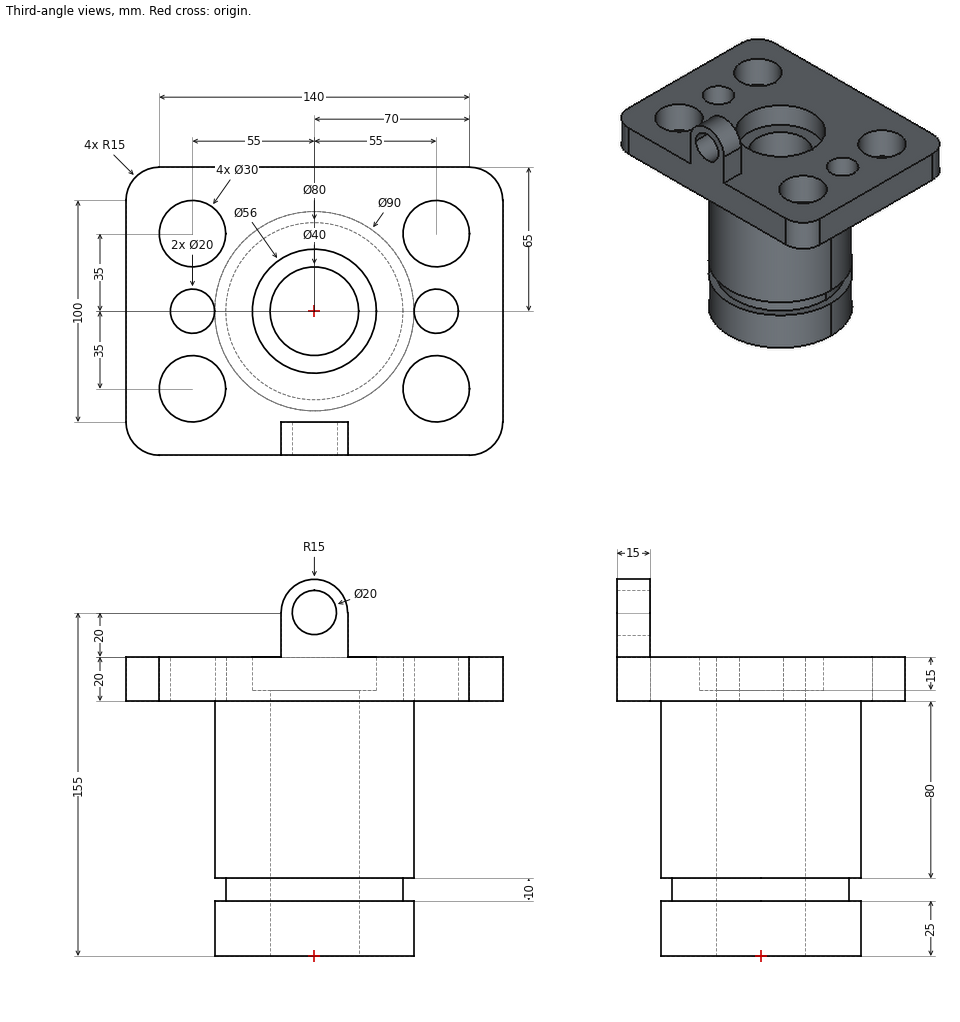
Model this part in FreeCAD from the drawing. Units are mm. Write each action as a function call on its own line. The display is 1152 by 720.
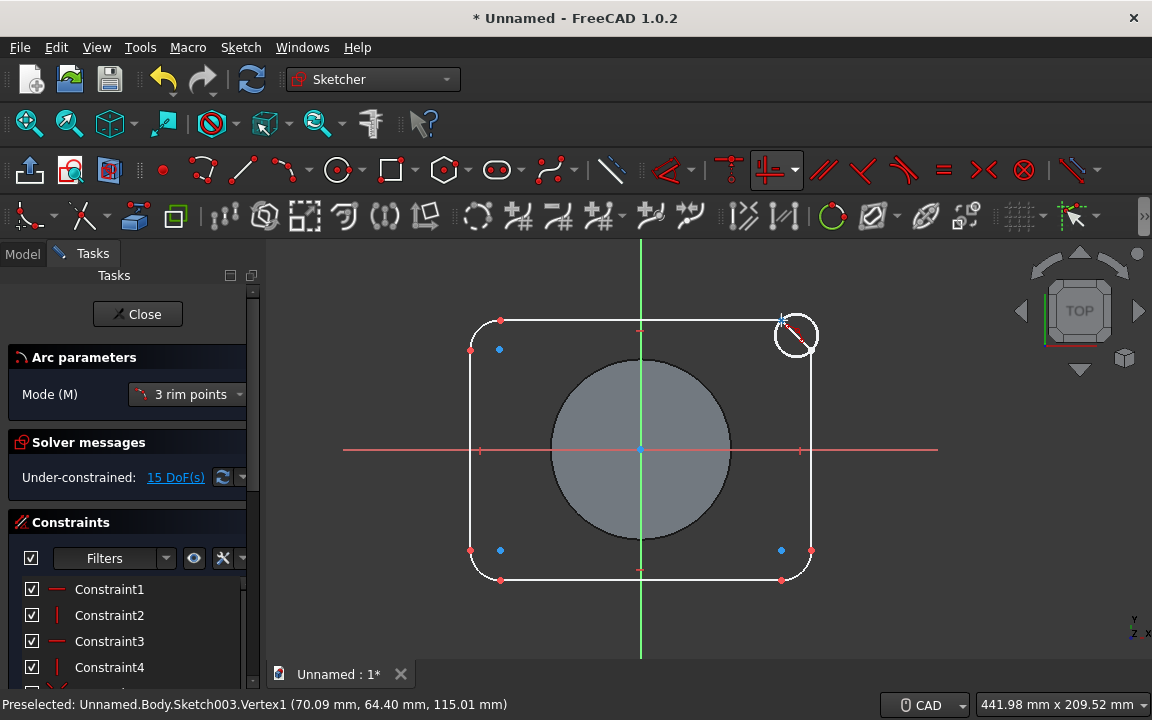
scroll(803, 328, up, 3)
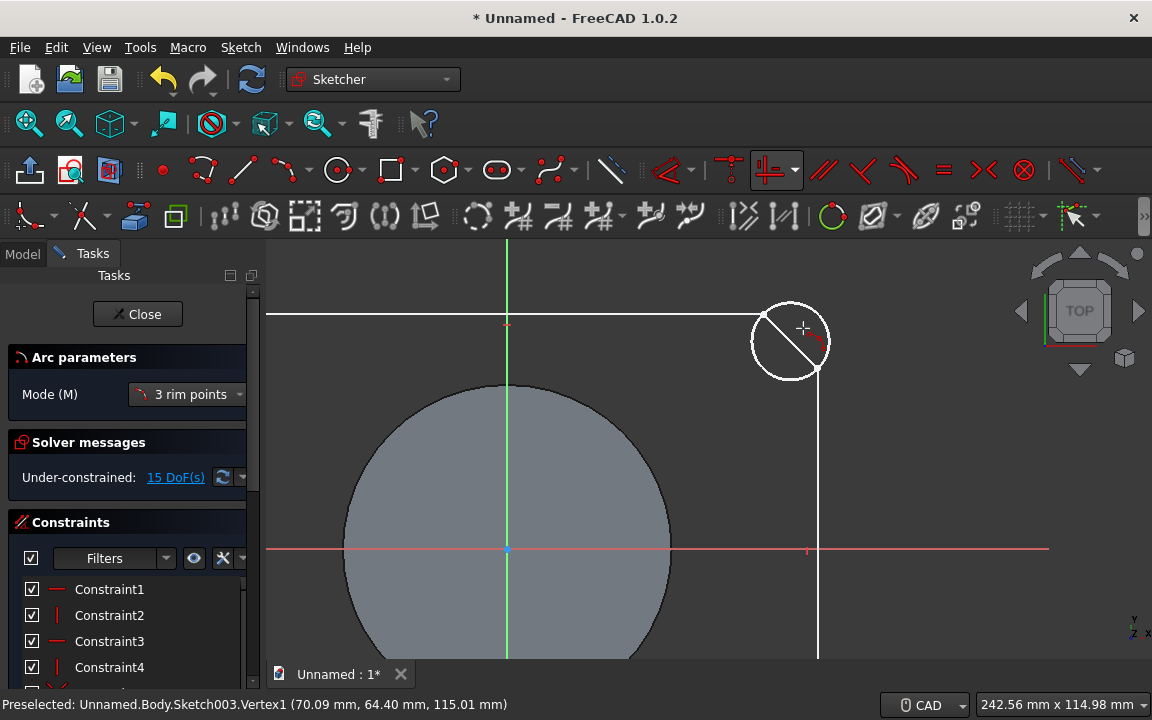
click(802, 328)
key(Escape)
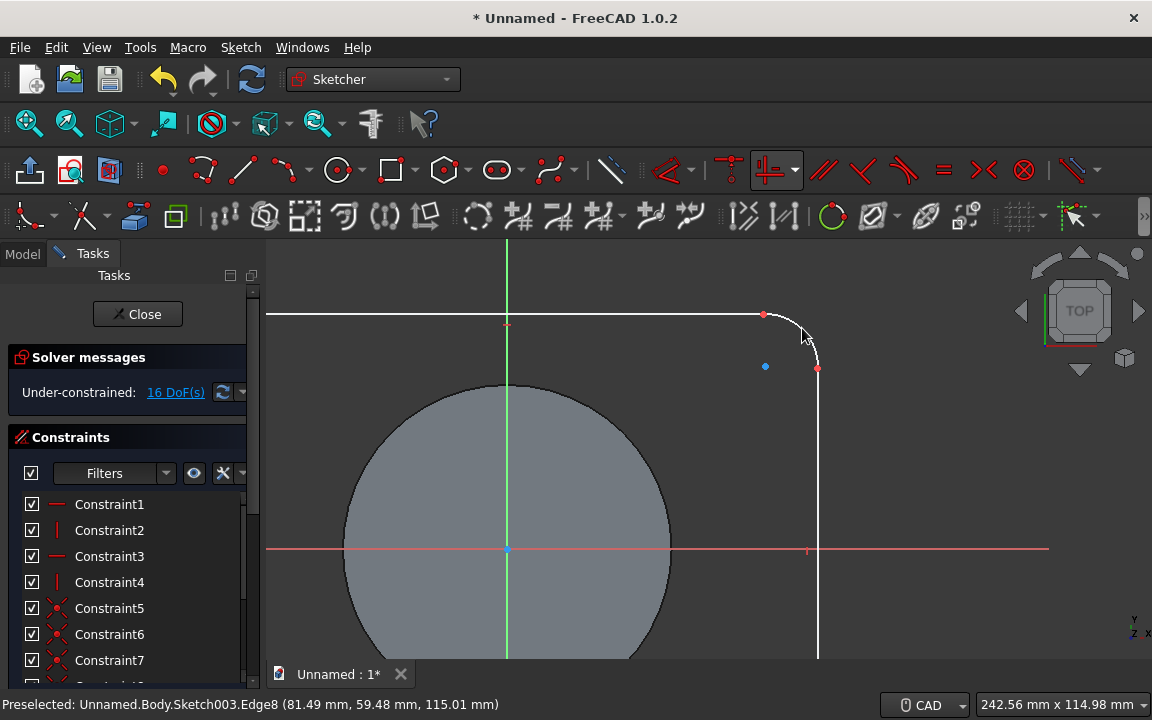
click(610, 314)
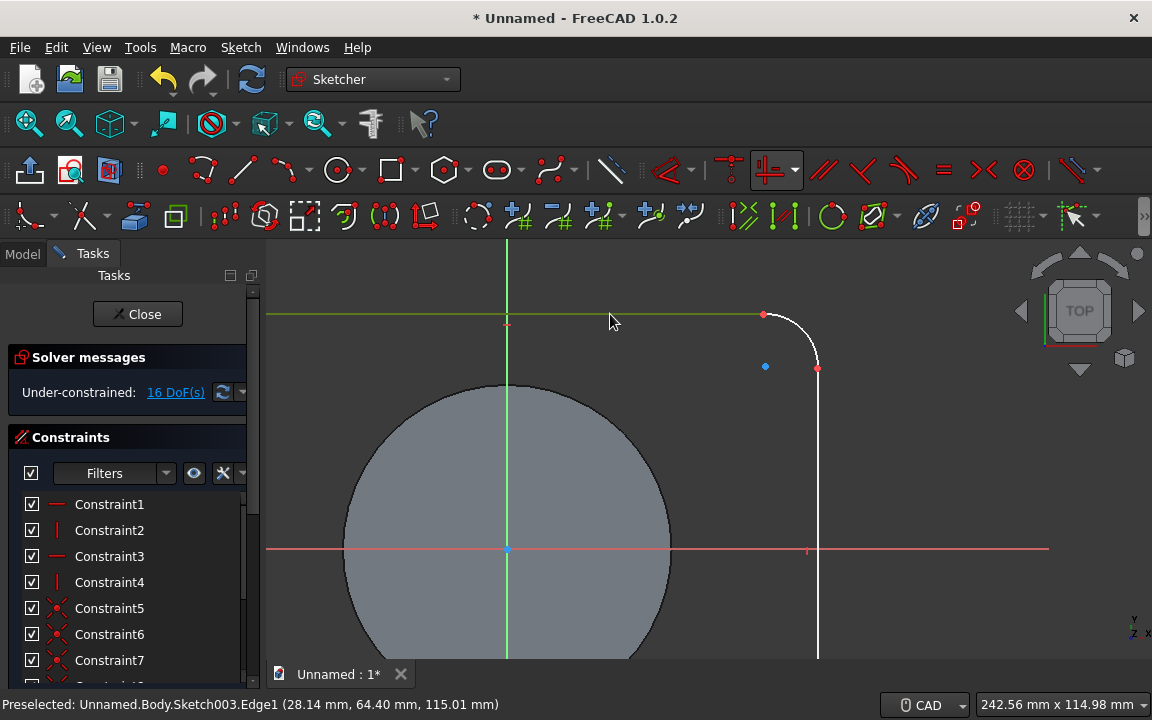
scroll(803, 327, down, 3)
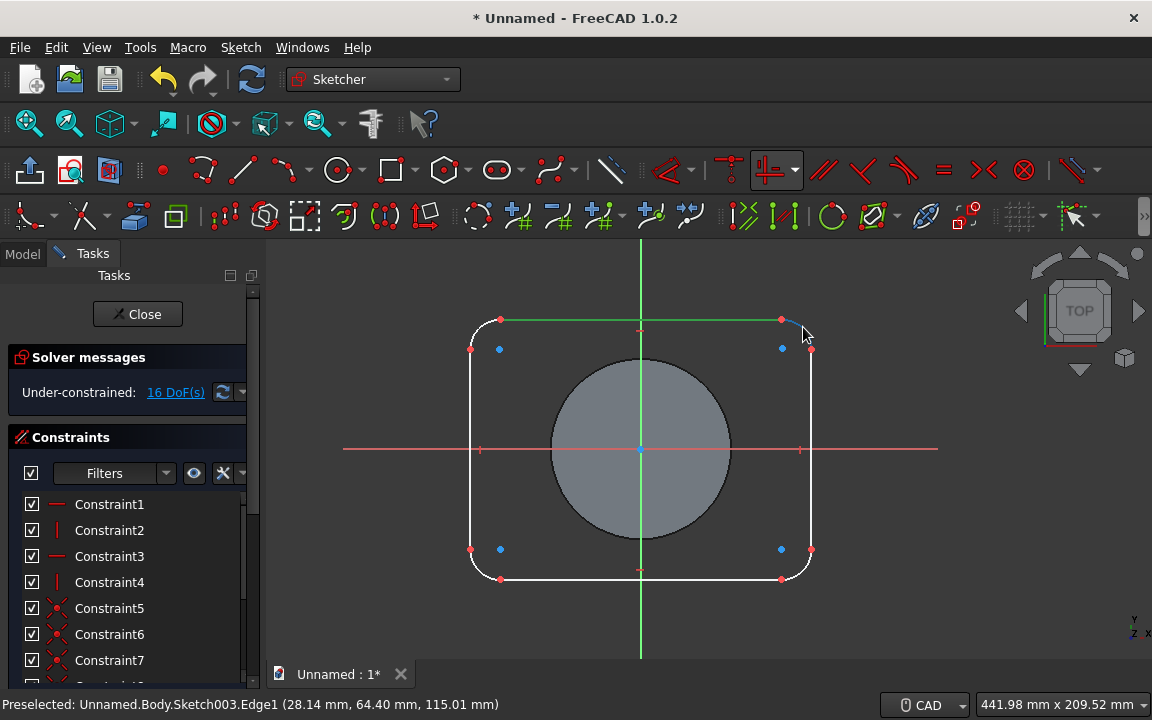
click(487, 323)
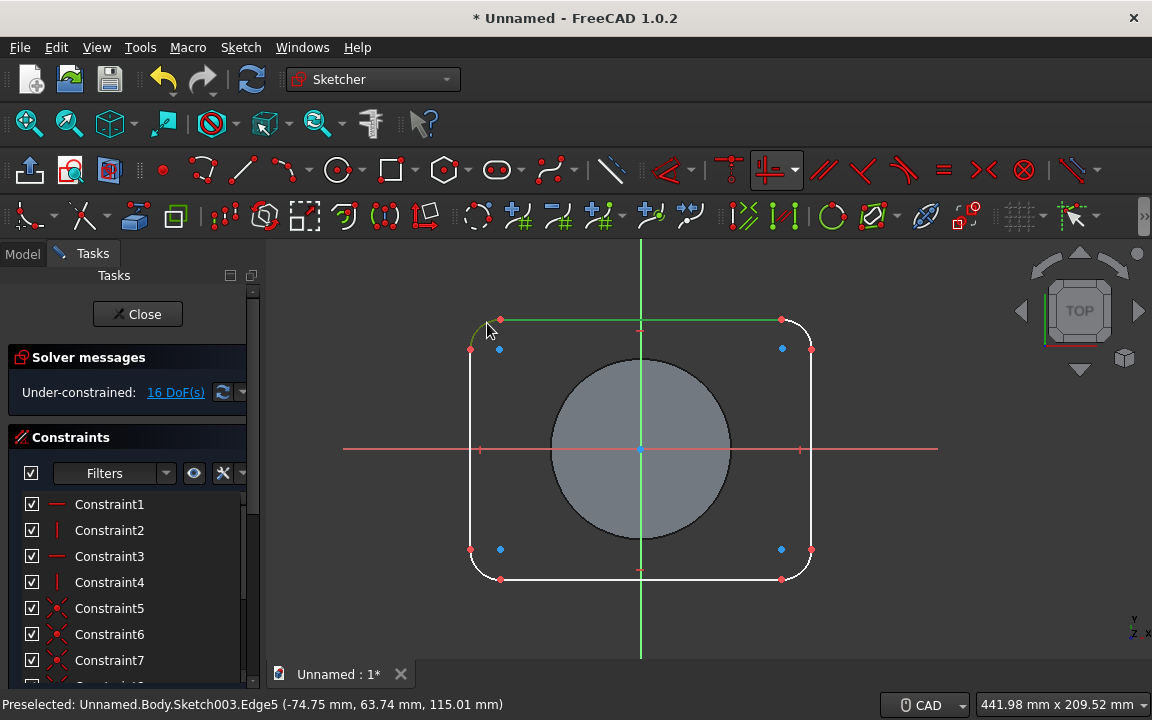
click(904, 170)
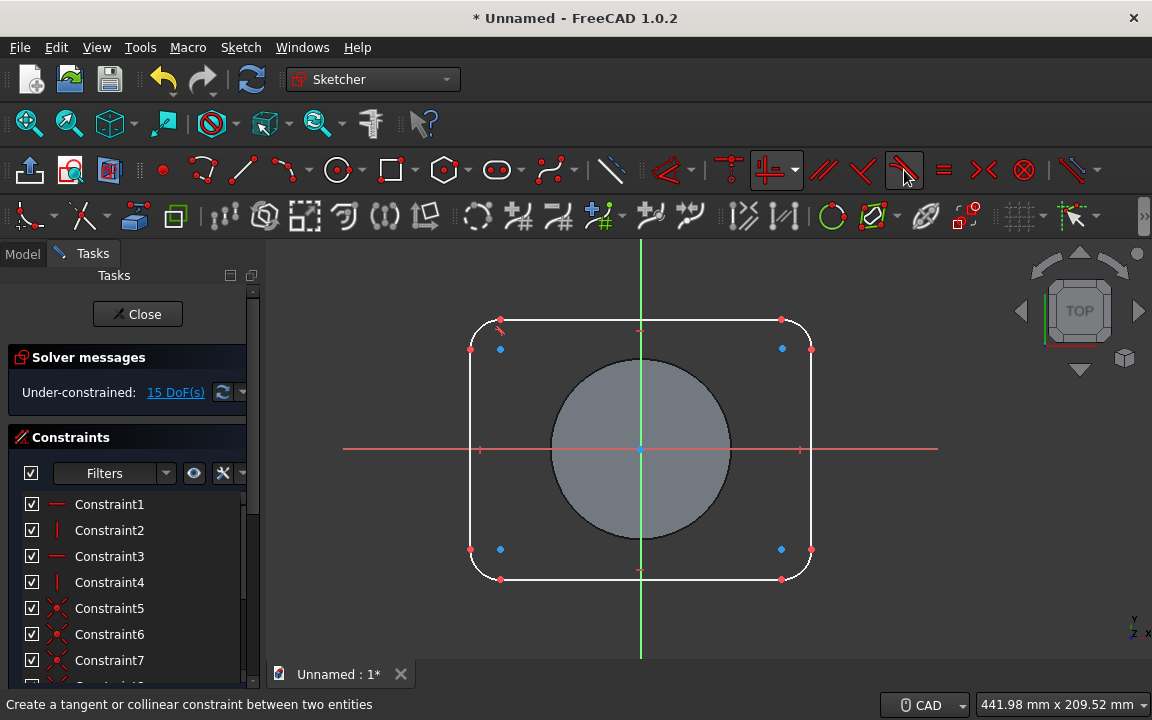
click(697, 320)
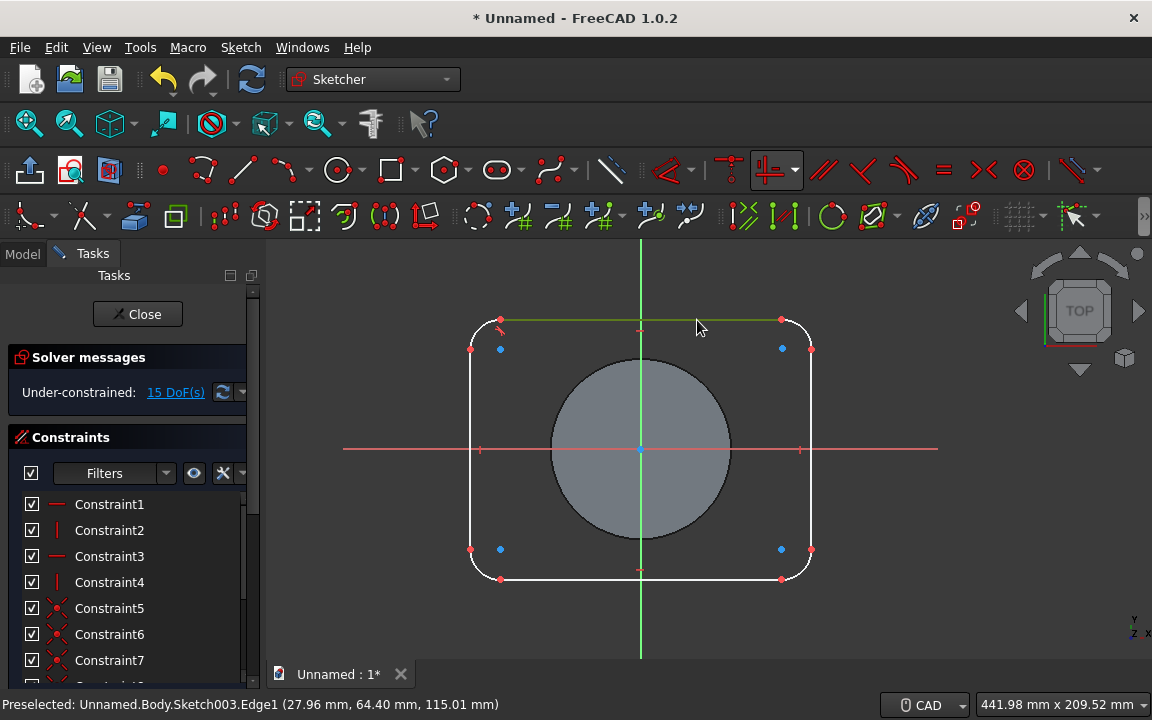
click(809, 336)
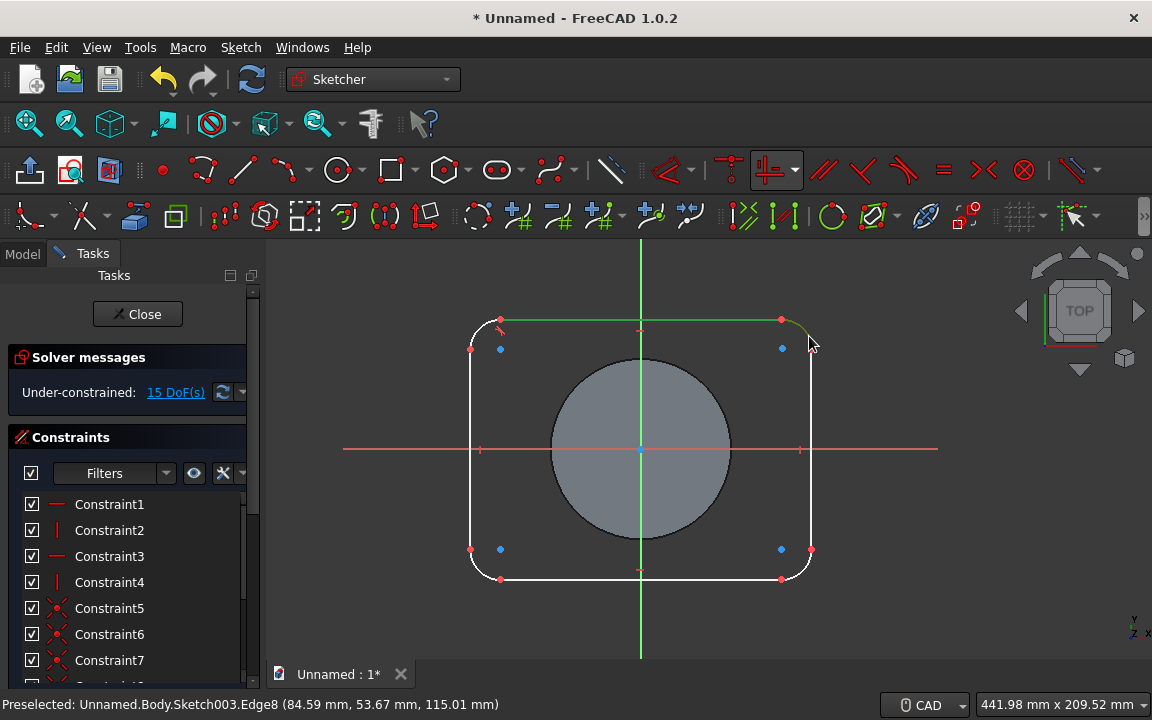
click(904, 170)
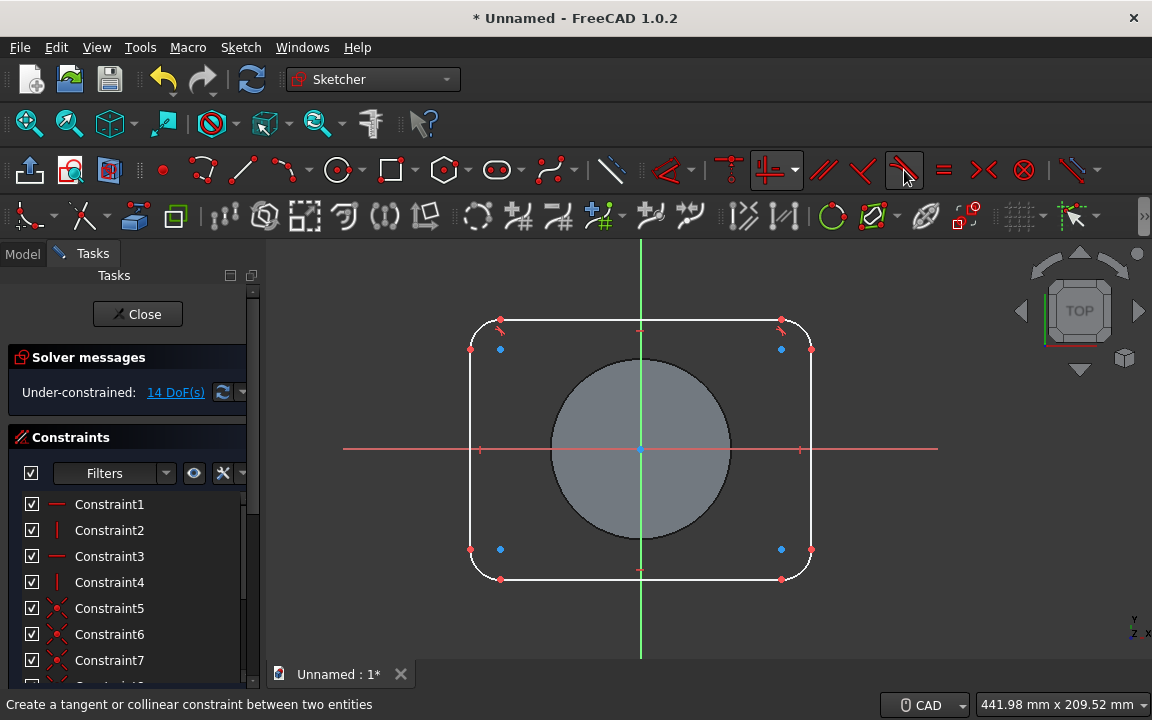
click(470, 410)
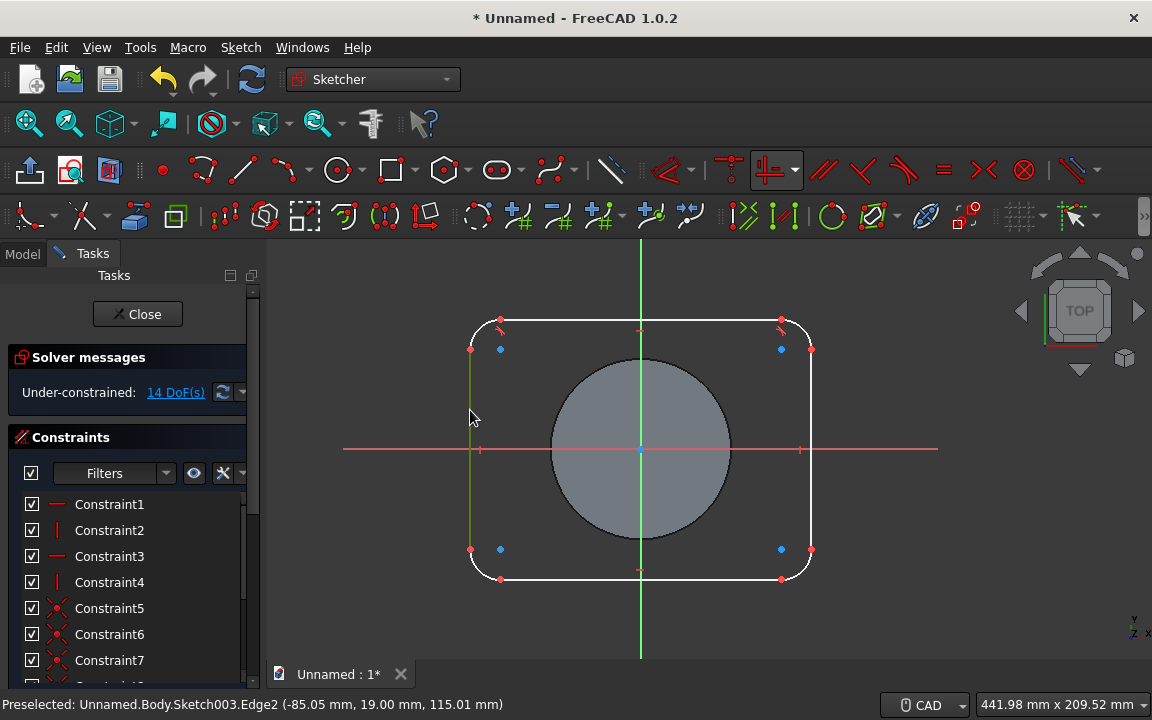
click(487, 323)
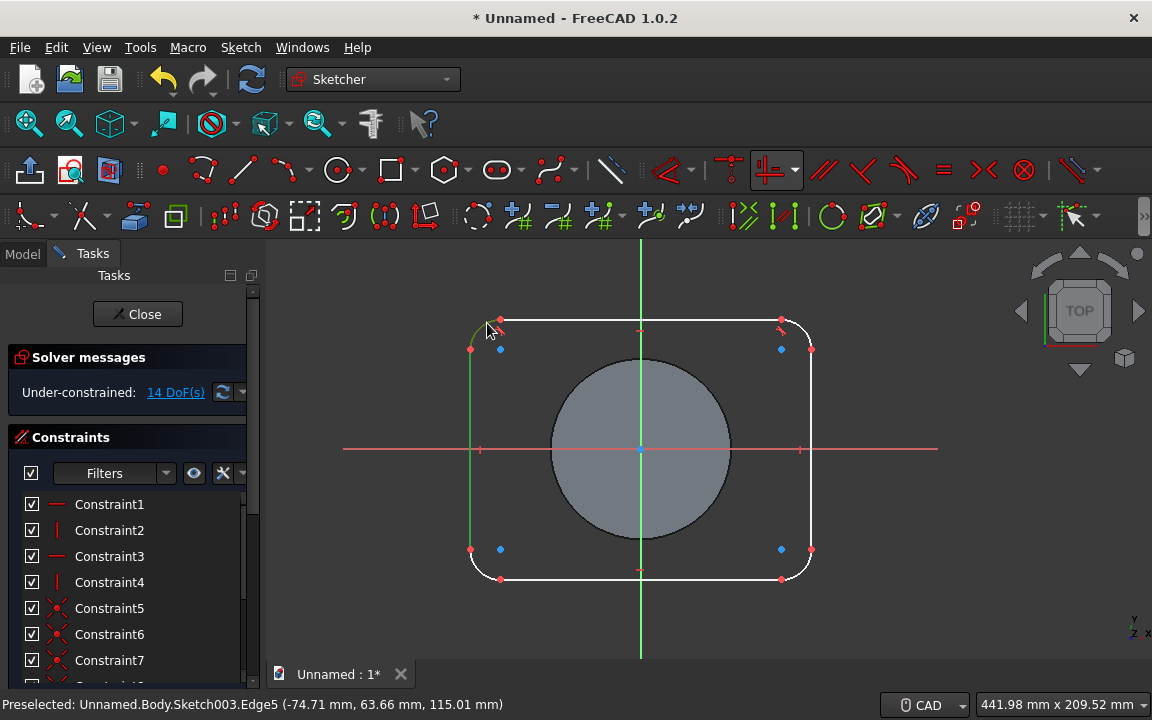
click(904, 170)